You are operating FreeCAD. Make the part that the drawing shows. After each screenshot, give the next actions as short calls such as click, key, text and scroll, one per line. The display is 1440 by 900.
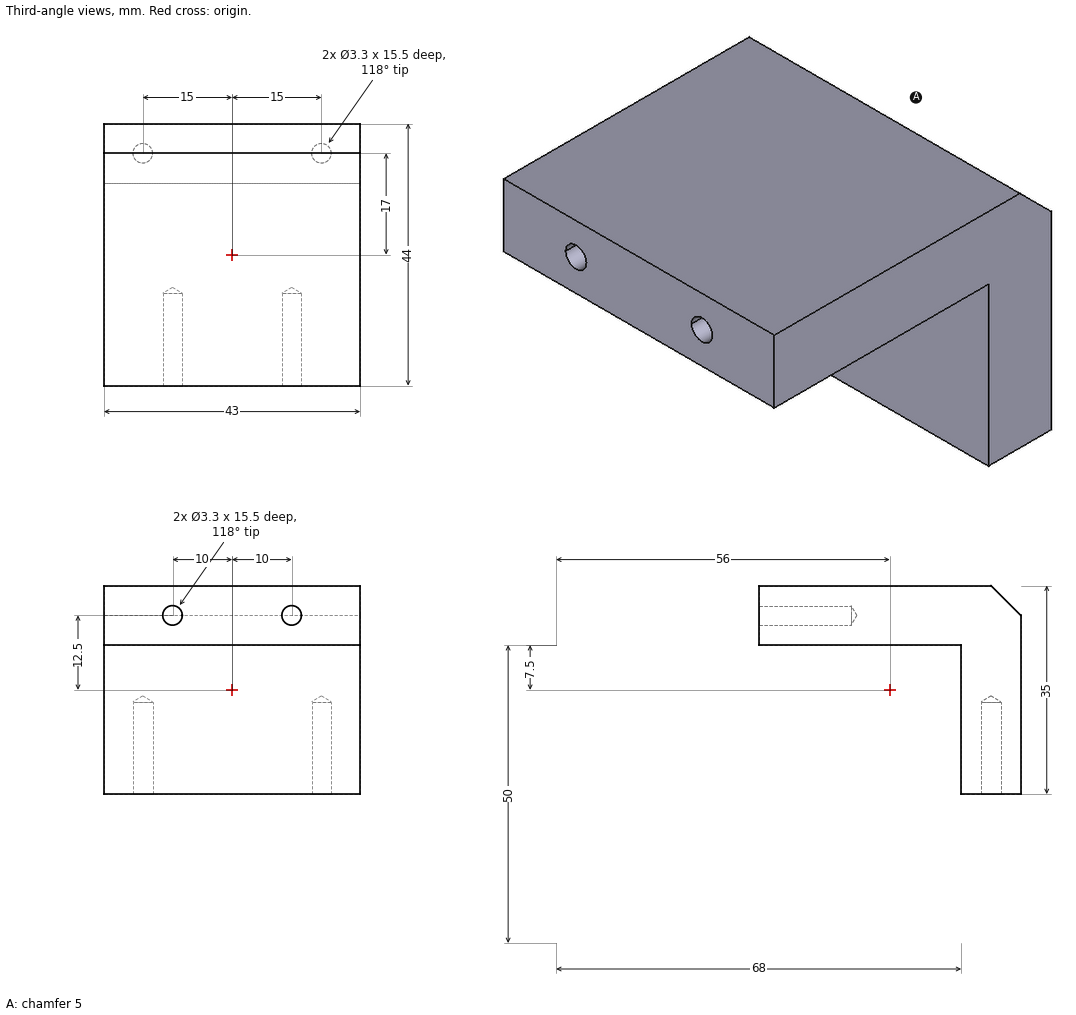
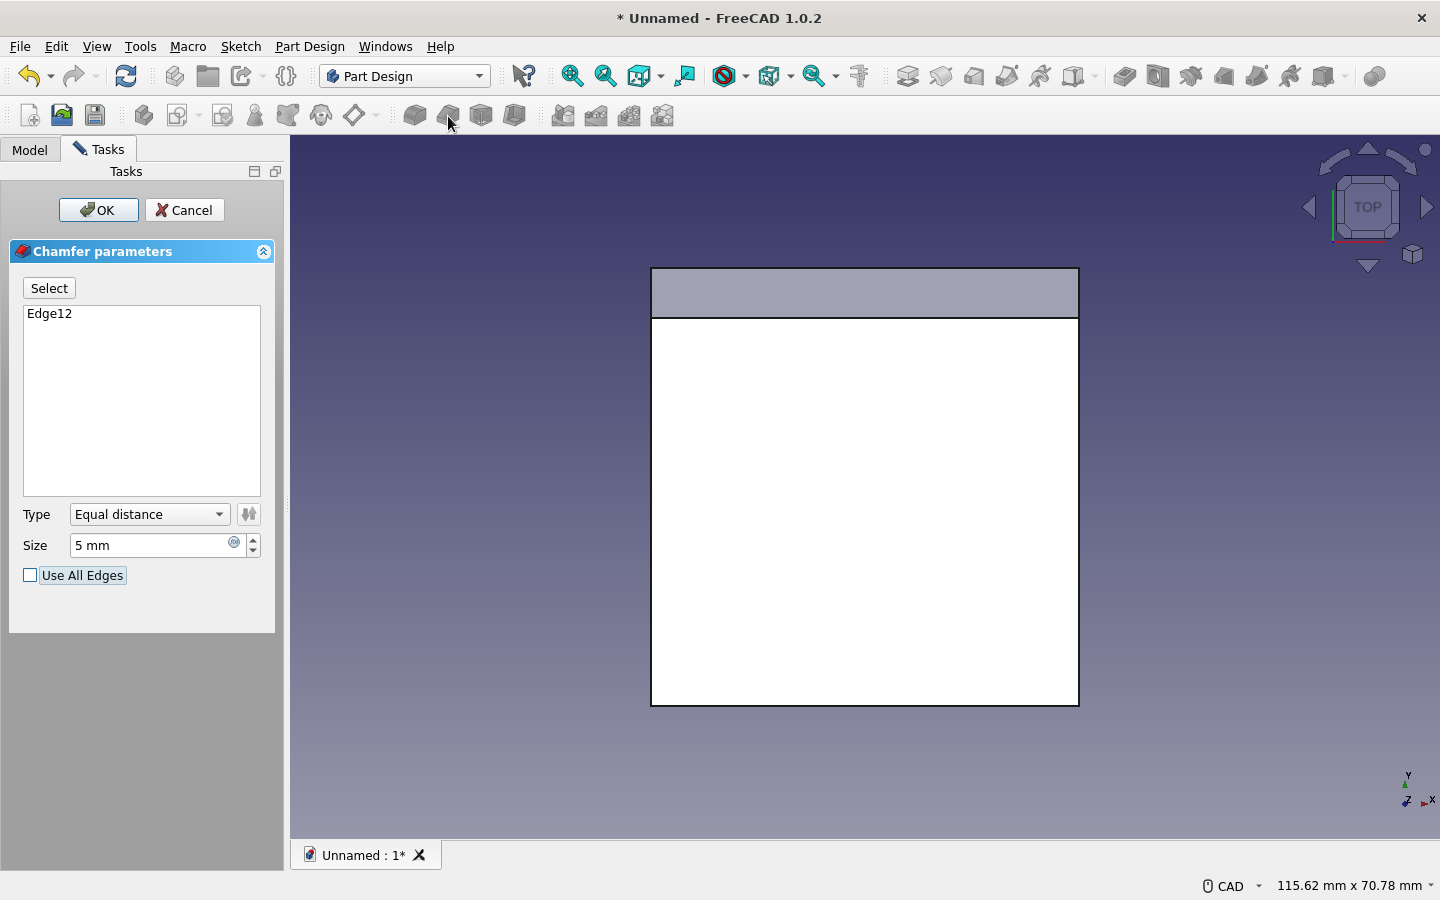
click(99, 210)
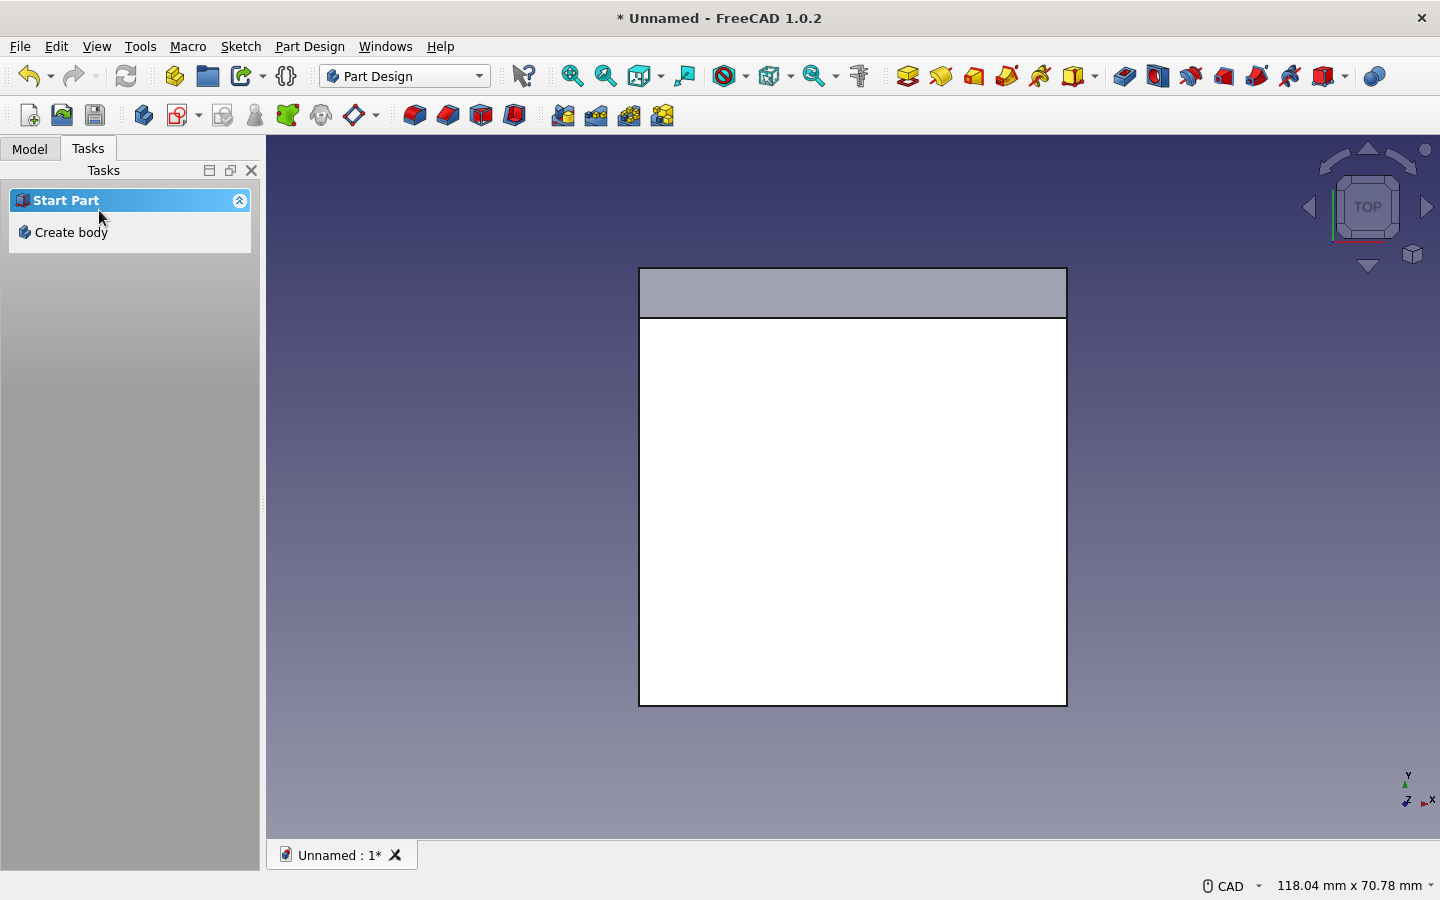
key(0)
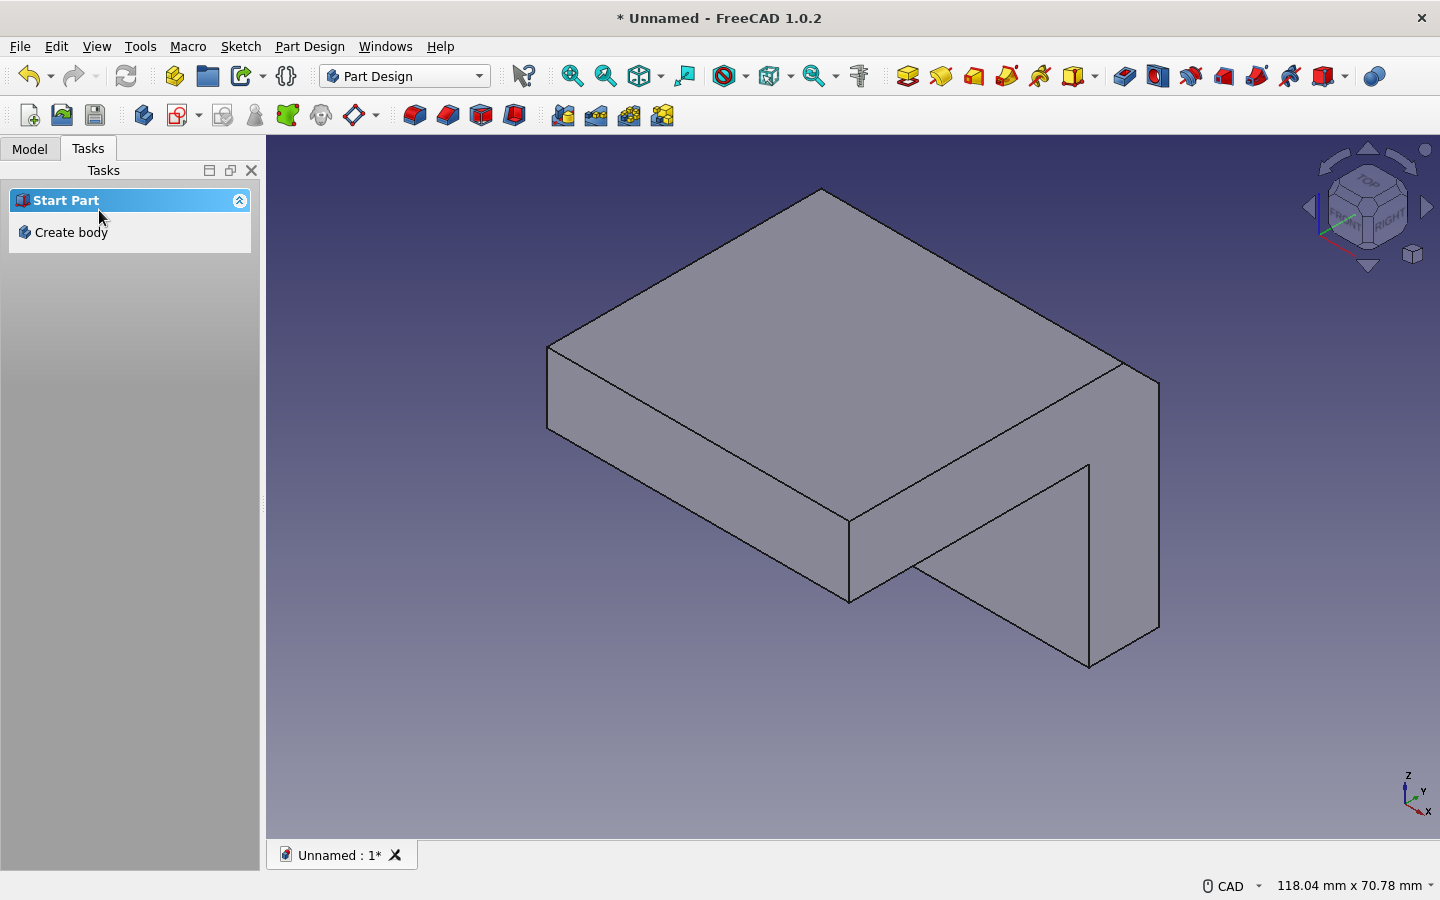
click(785, 524)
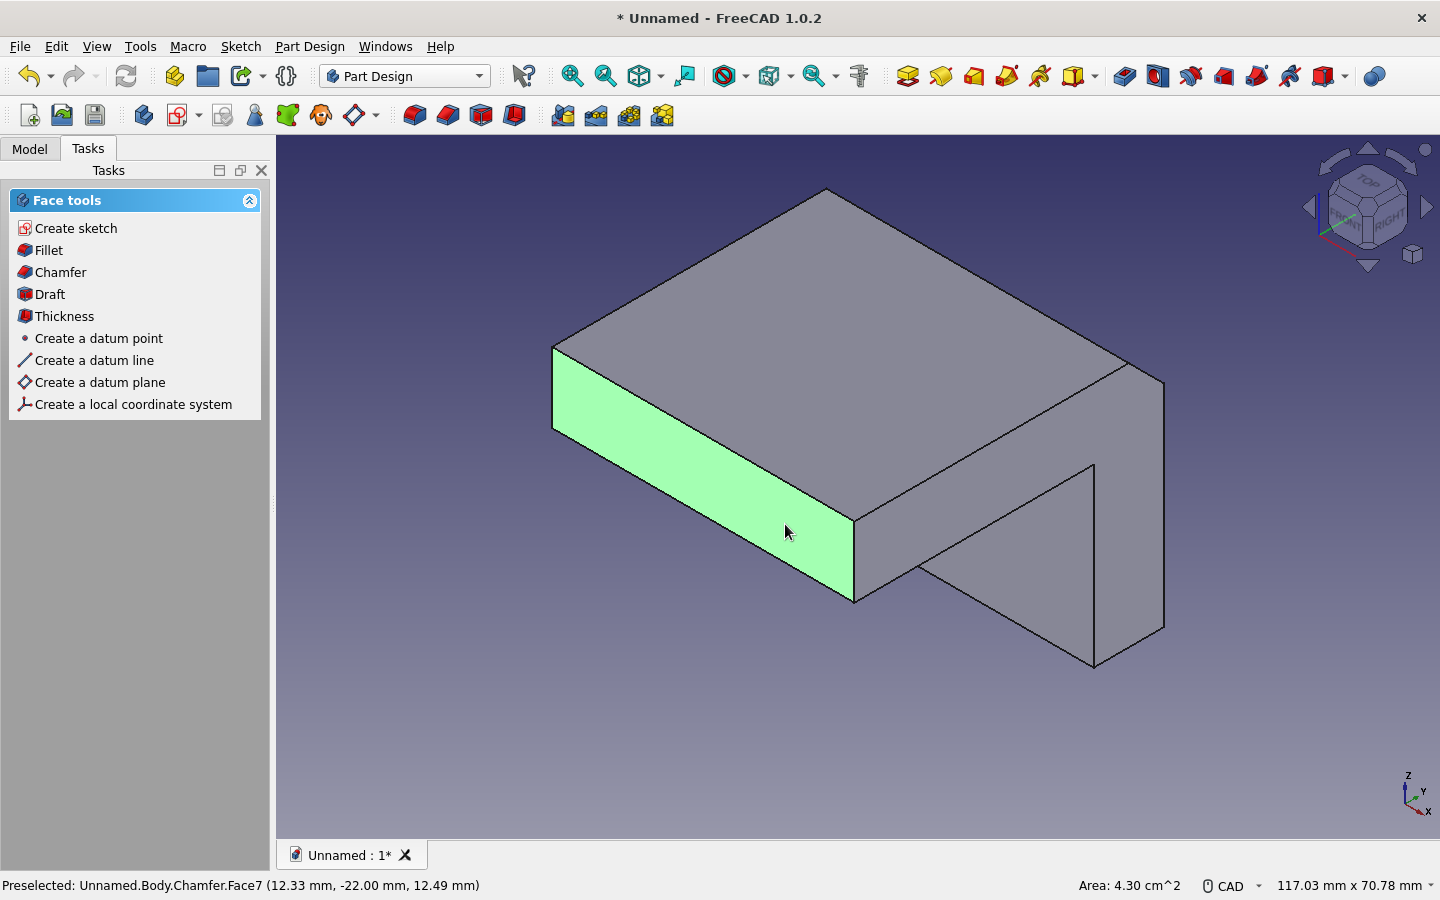
click(176, 116)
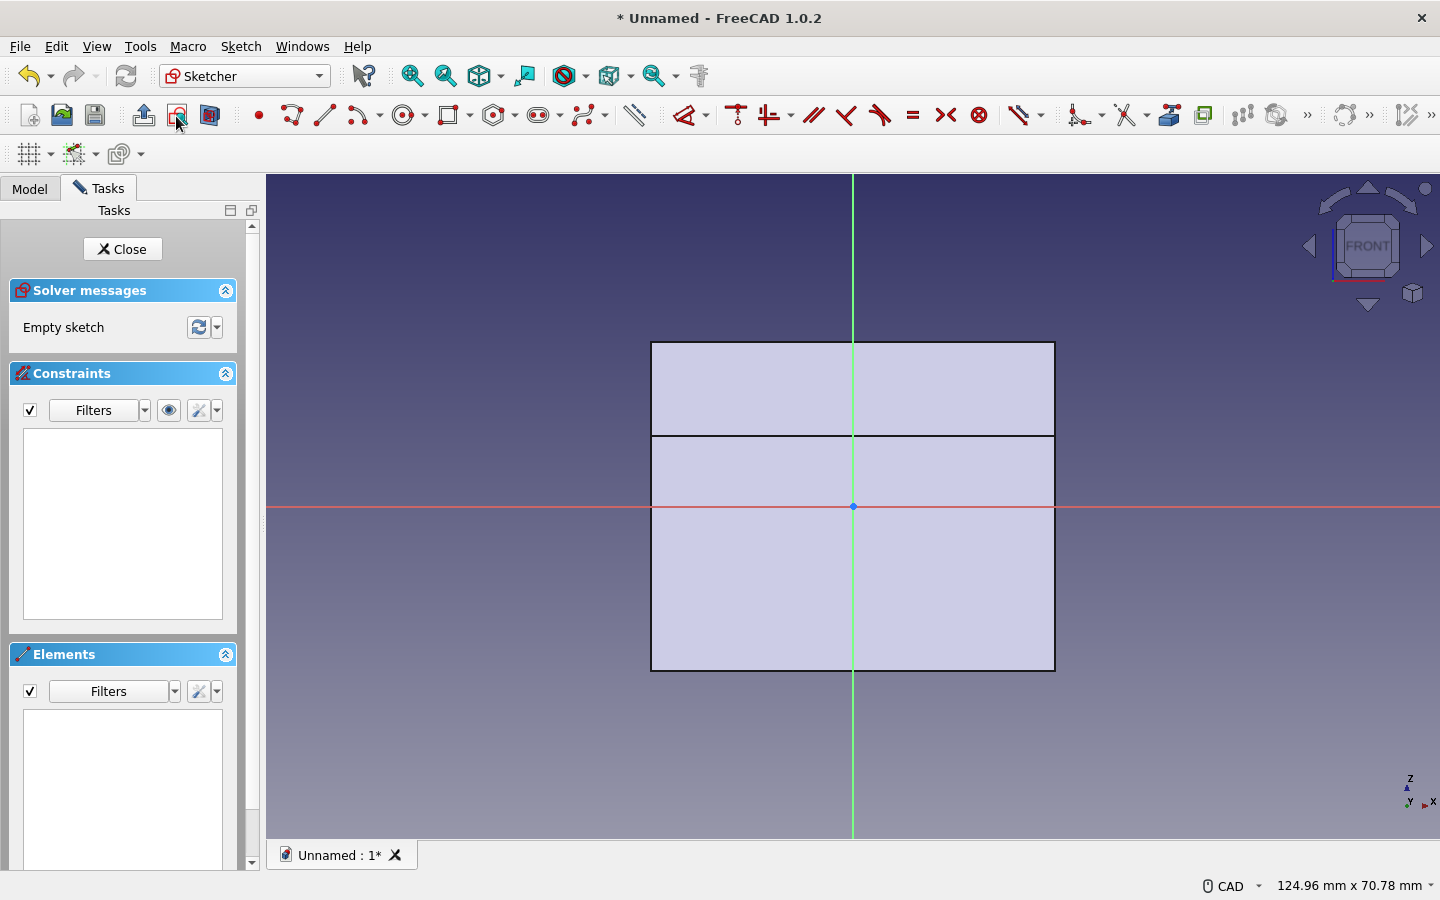
scroll(883, 411, up, 6)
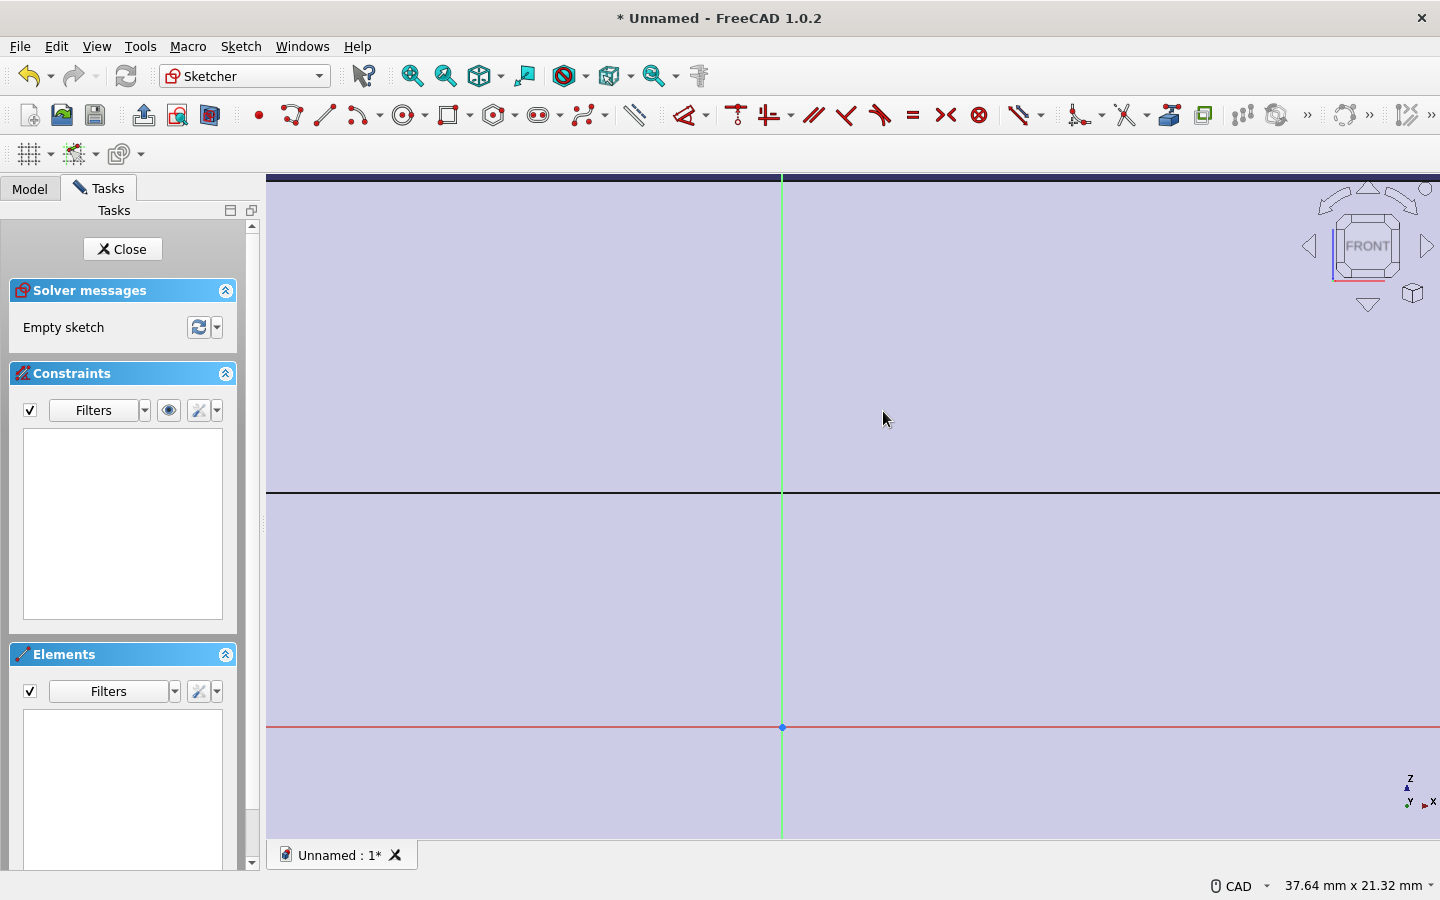
click(402, 116)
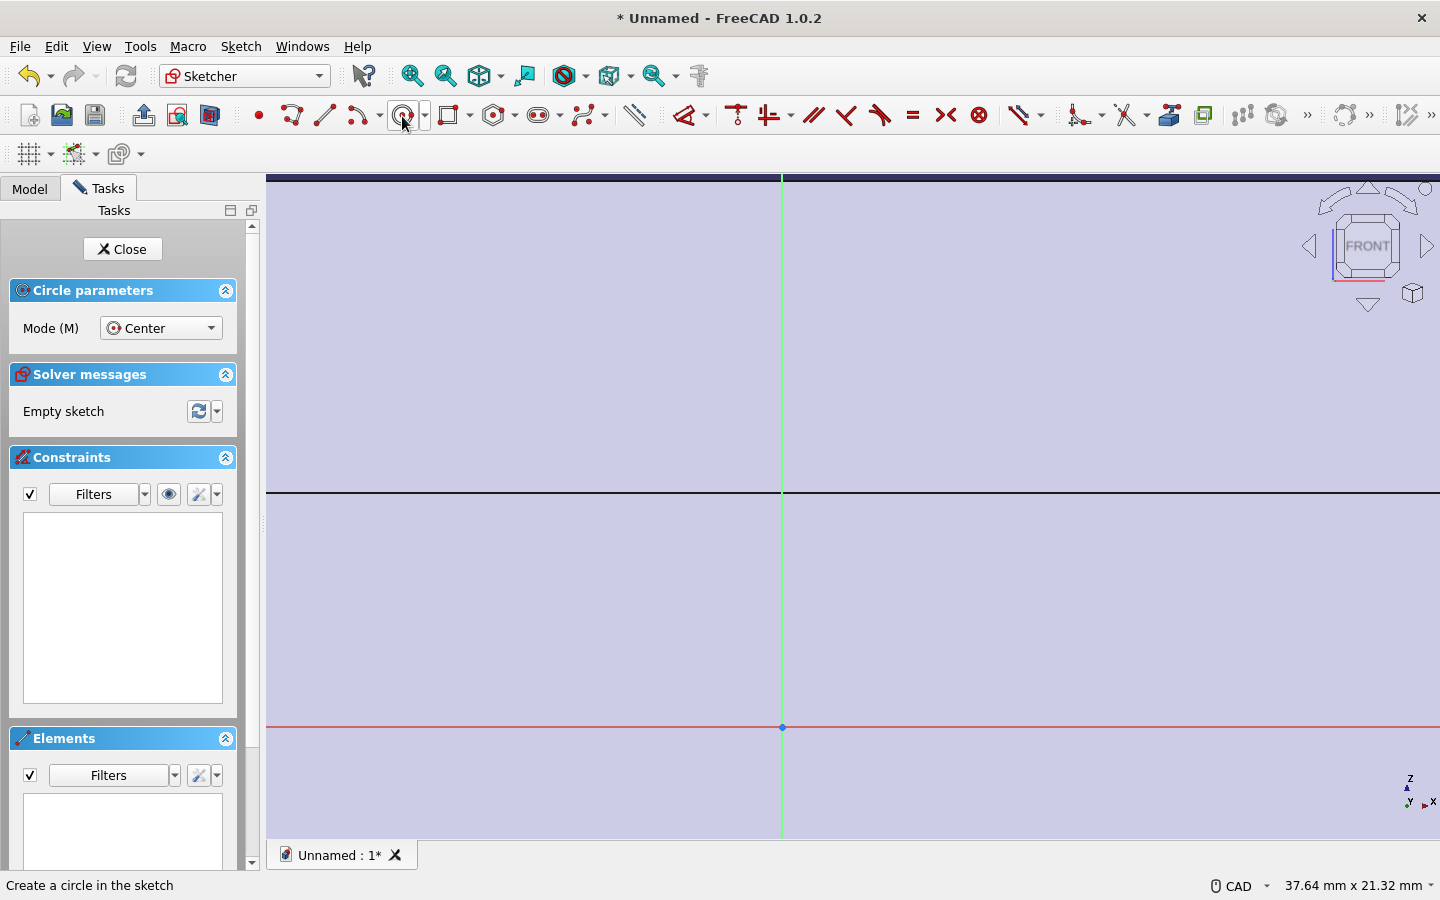
click(470, 337)
click(507, 301)